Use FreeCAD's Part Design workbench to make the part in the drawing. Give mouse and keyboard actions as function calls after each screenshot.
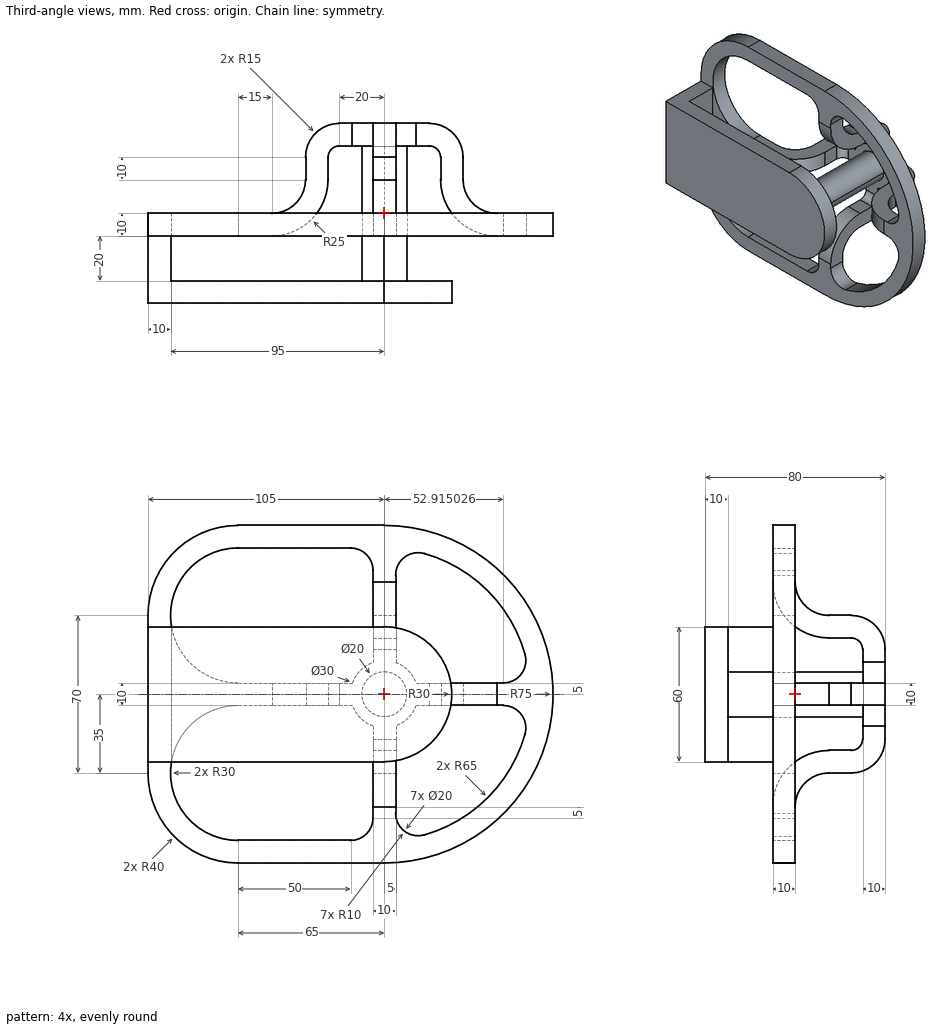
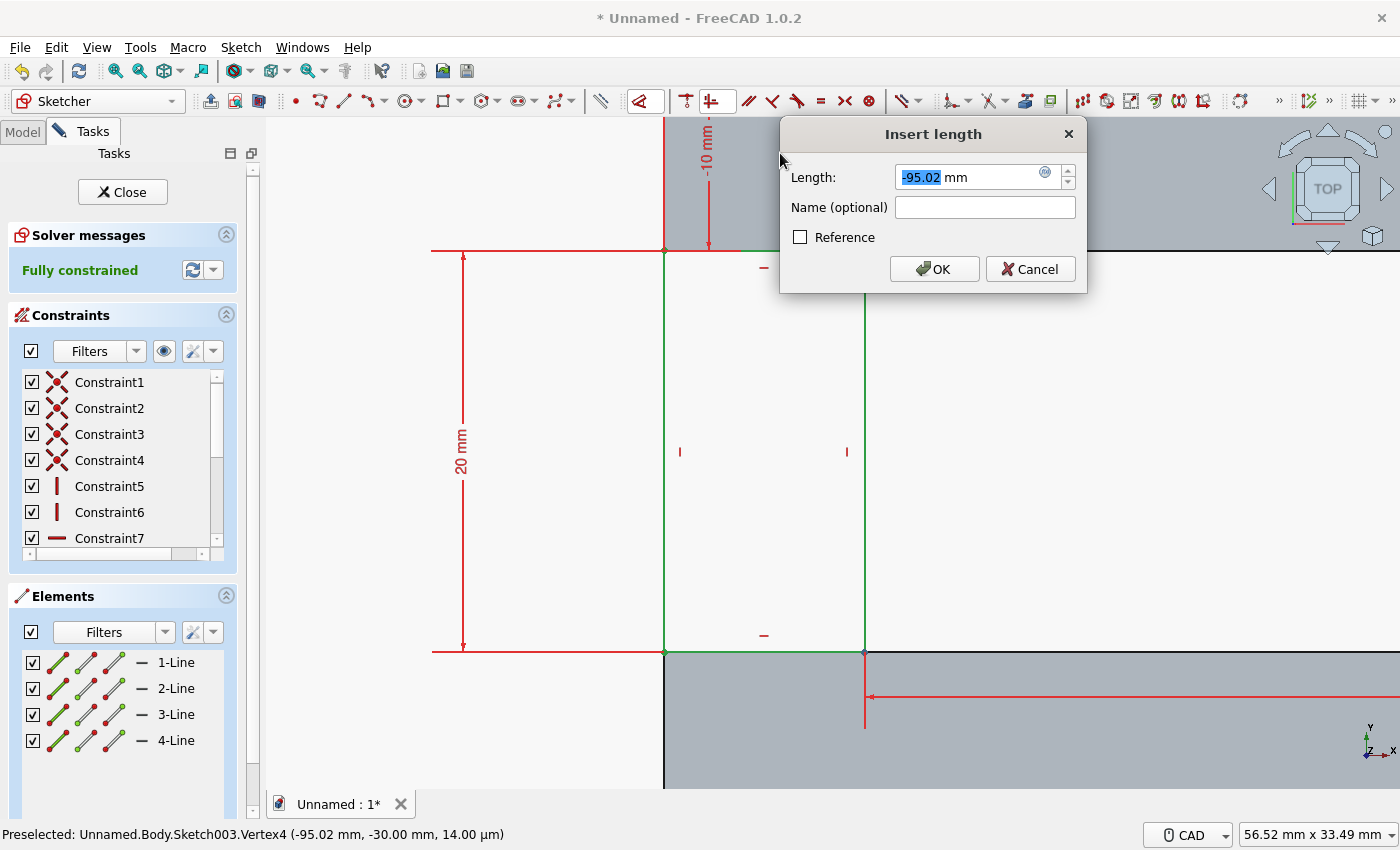
text(-95)
key(Return)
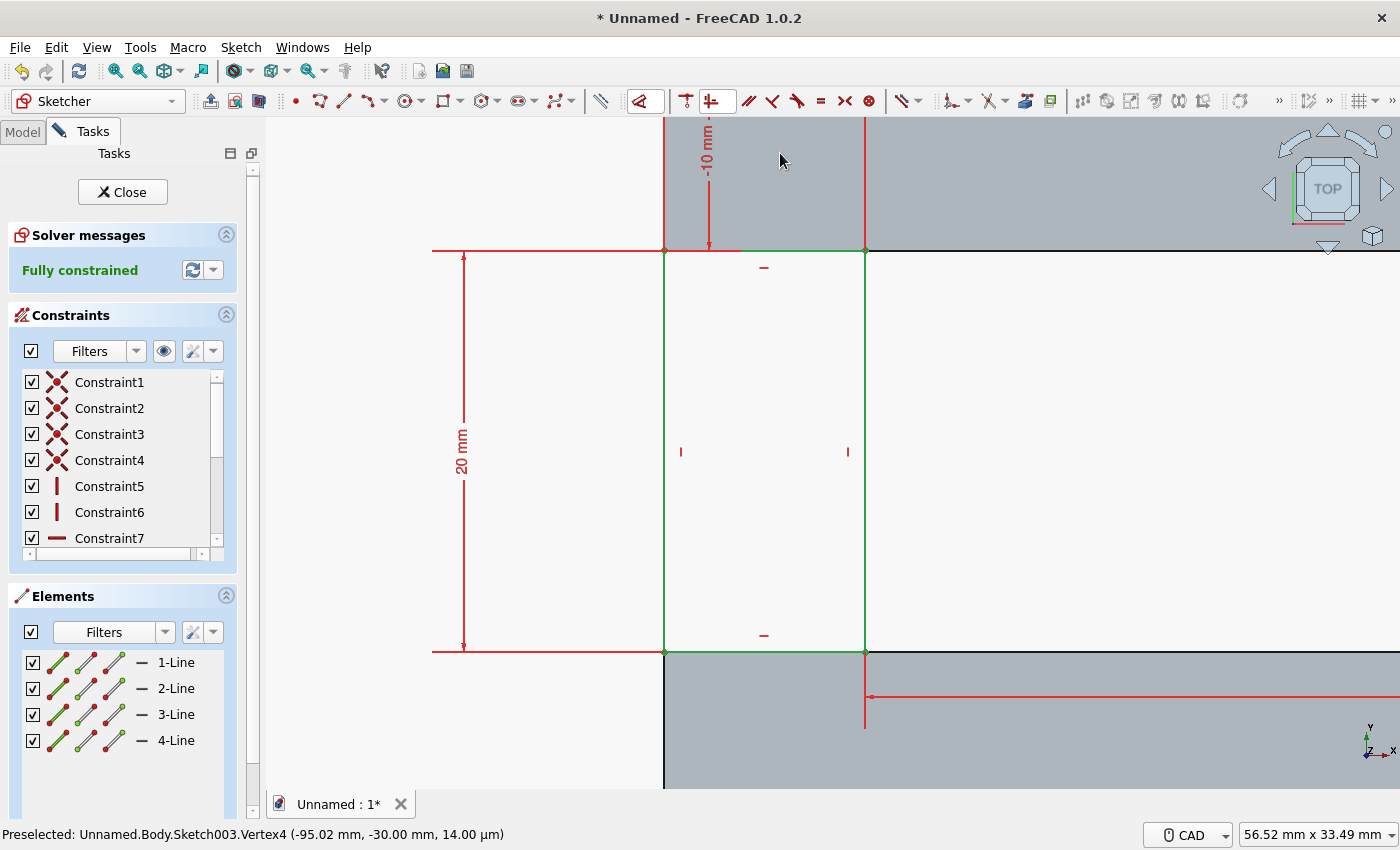
click(123, 192)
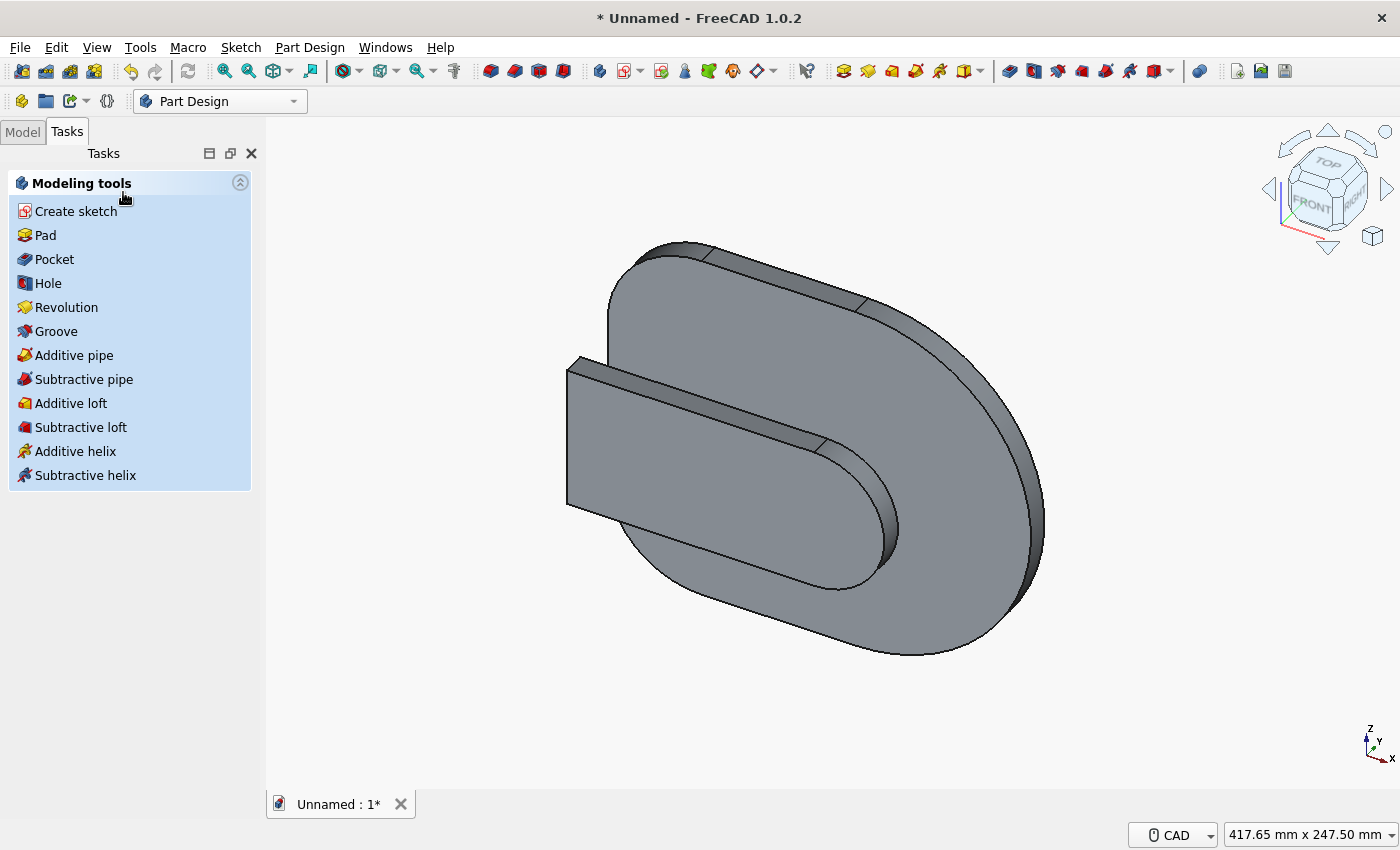
click(844, 72)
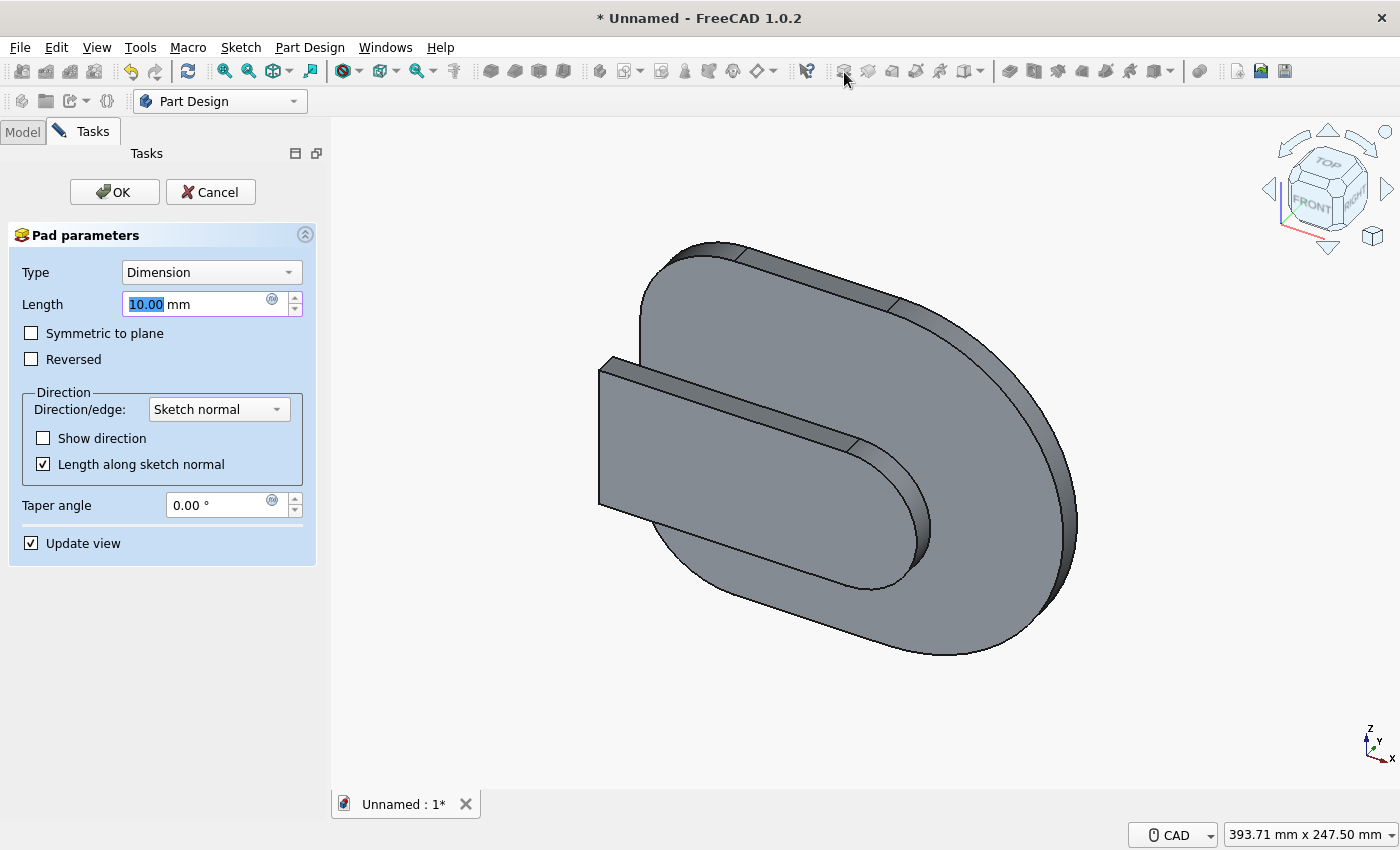
text(60)
key(Tab)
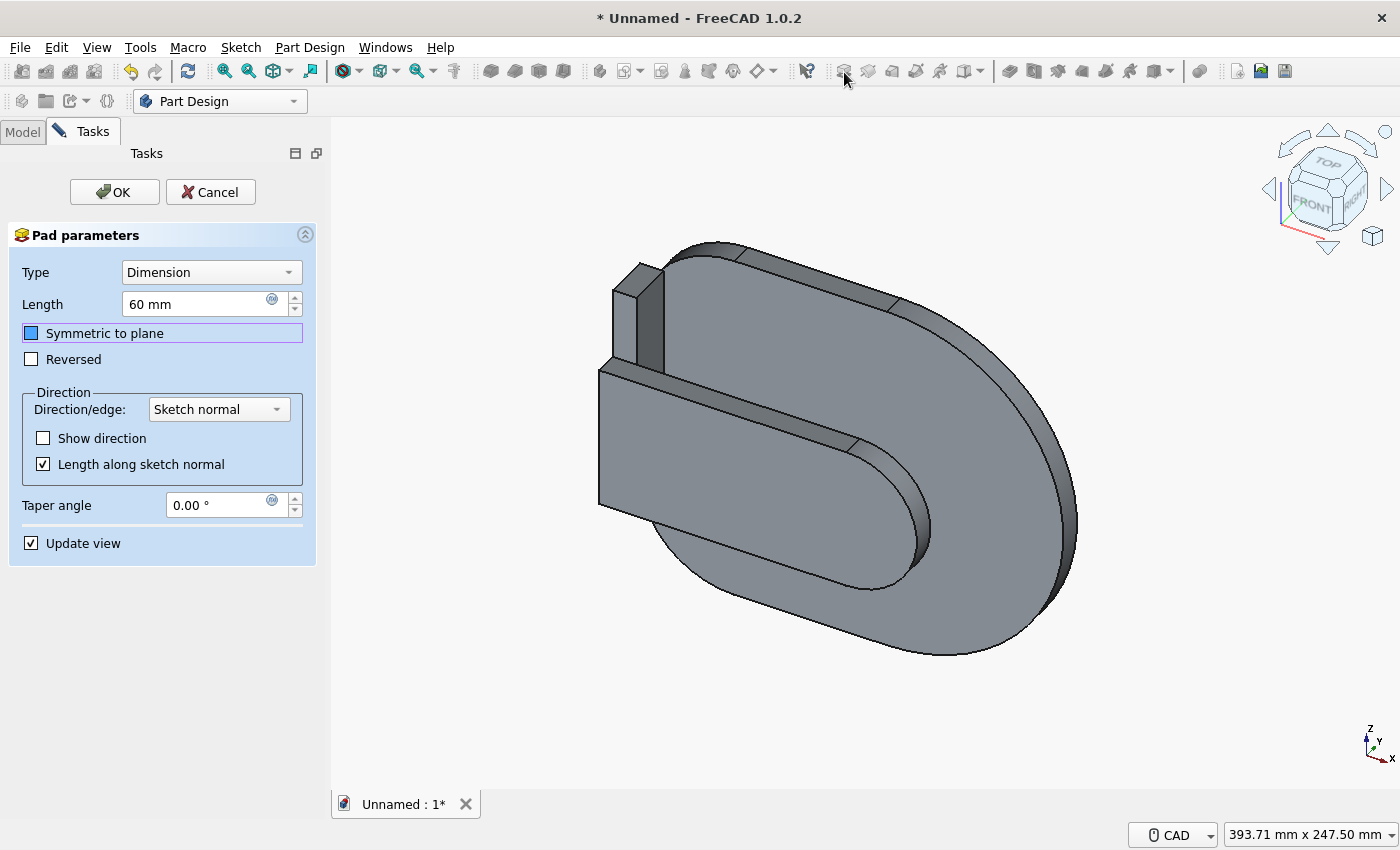
click(30, 333)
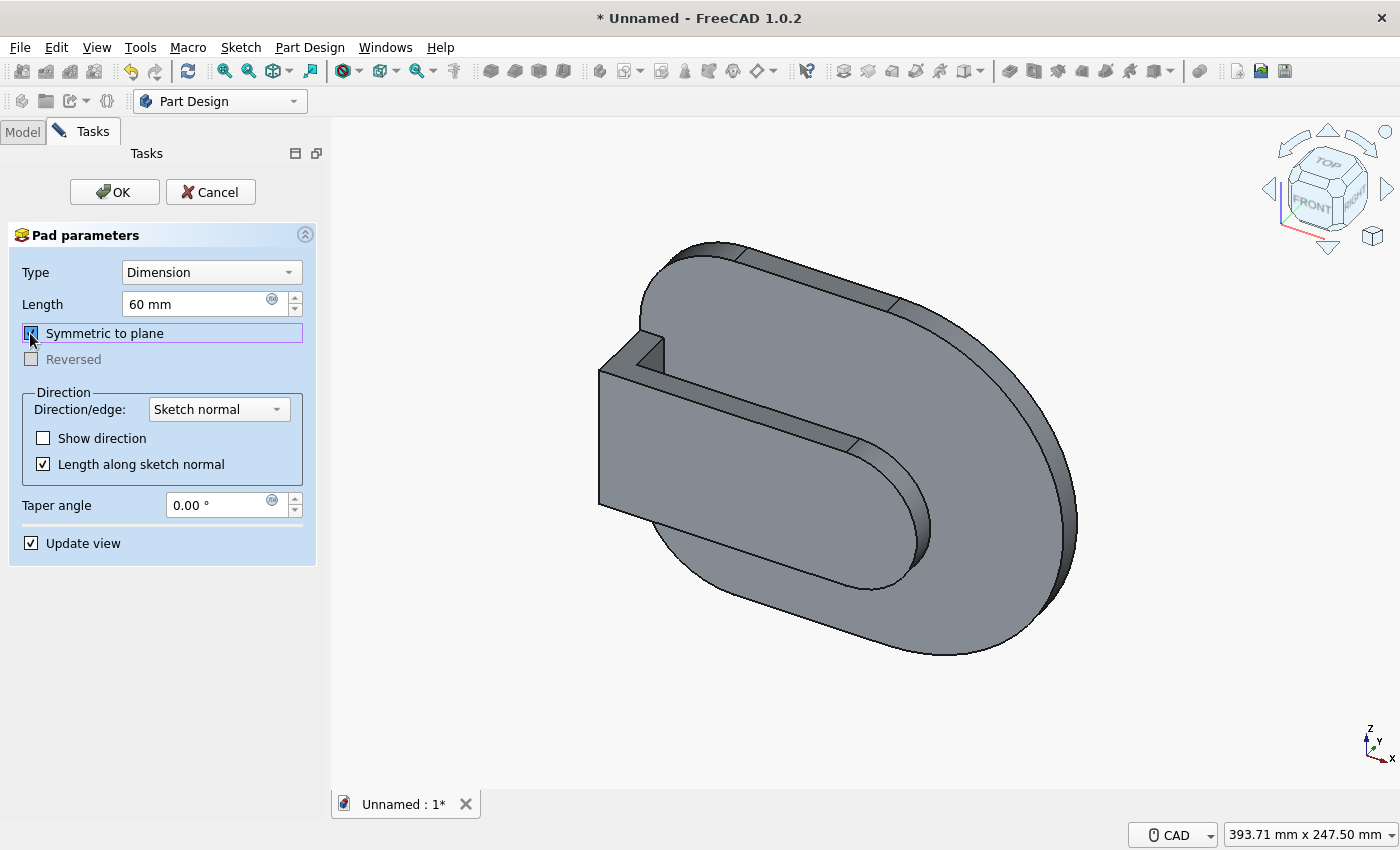
click(115, 192)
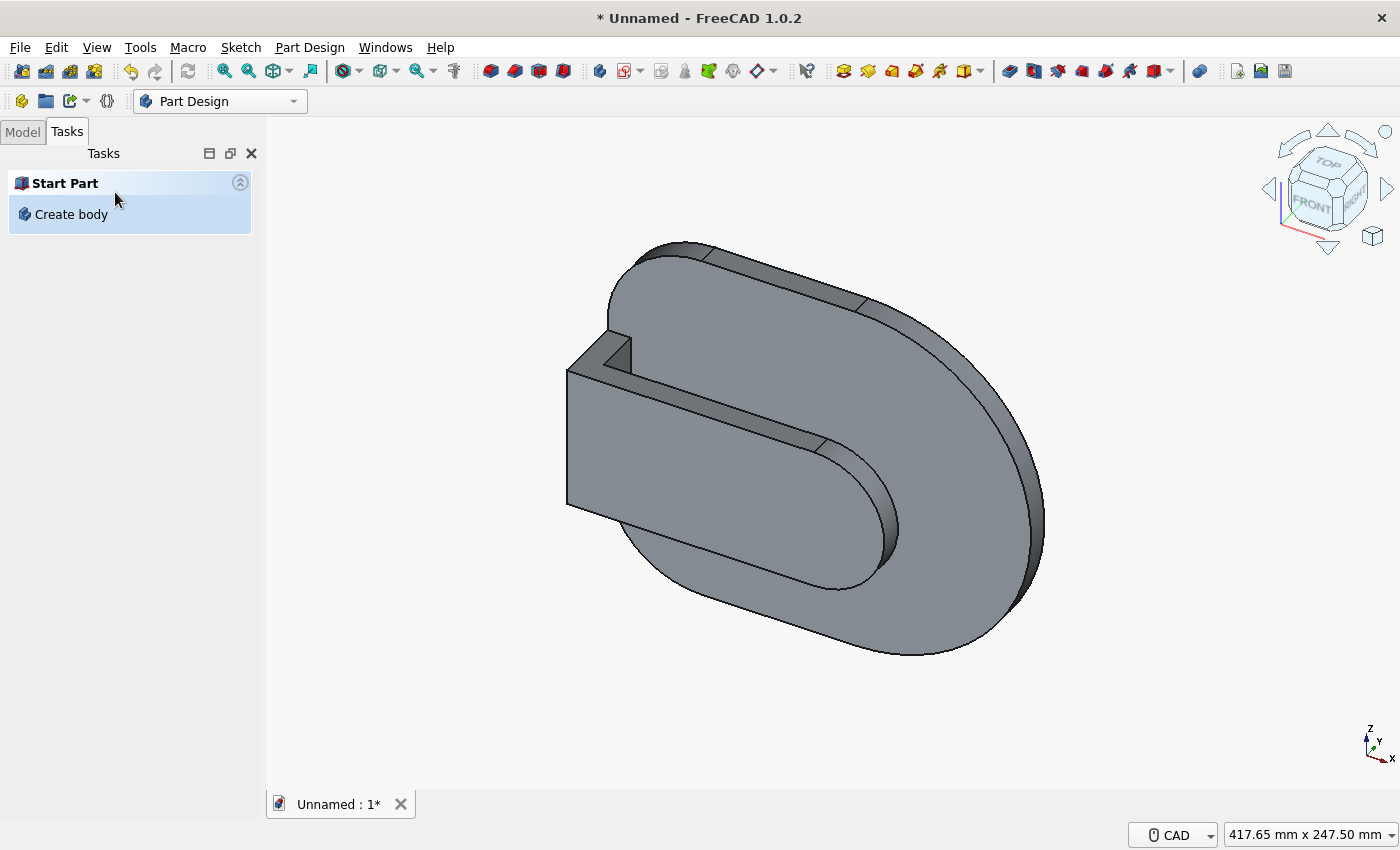
key(4)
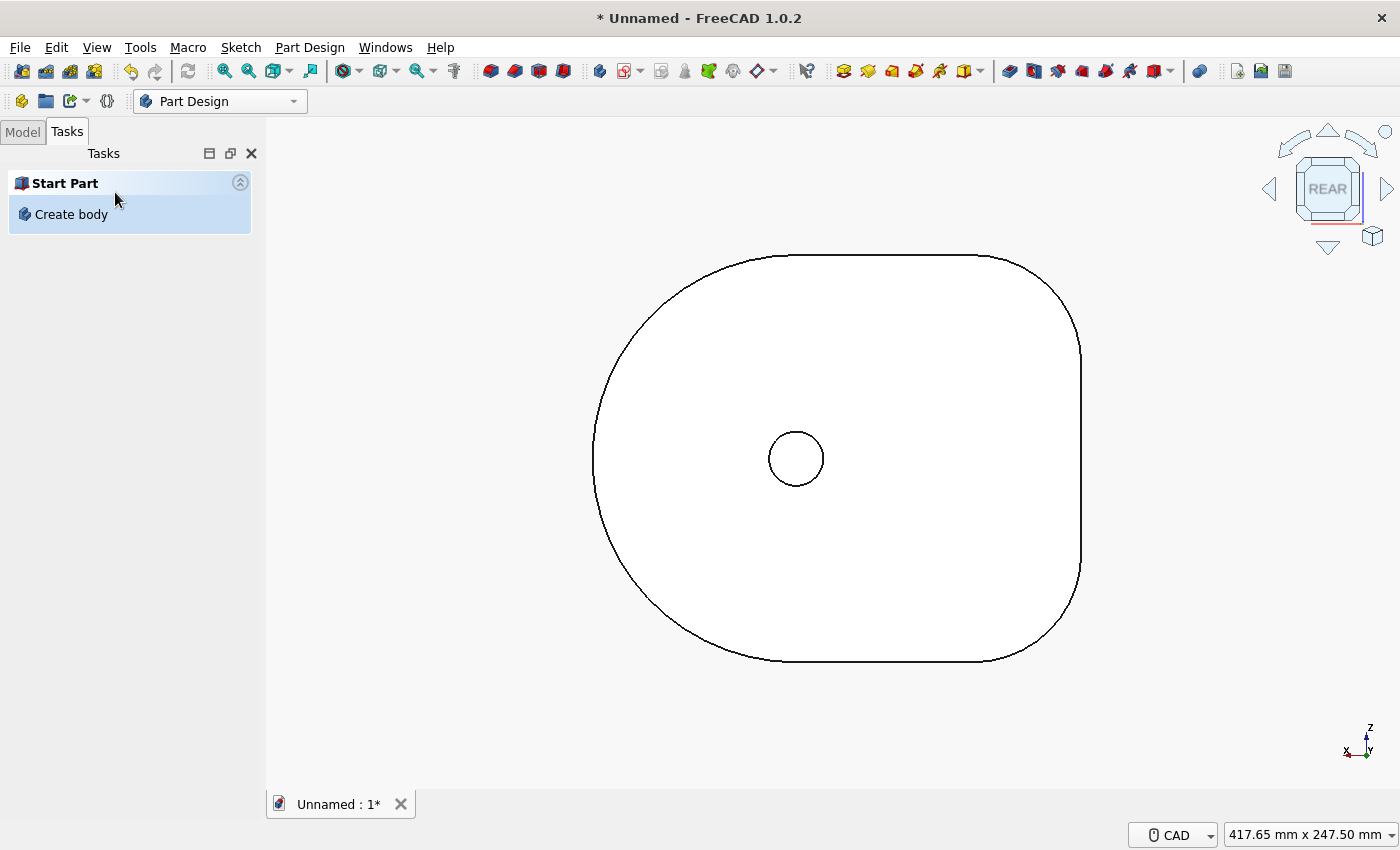
click(796, 458)